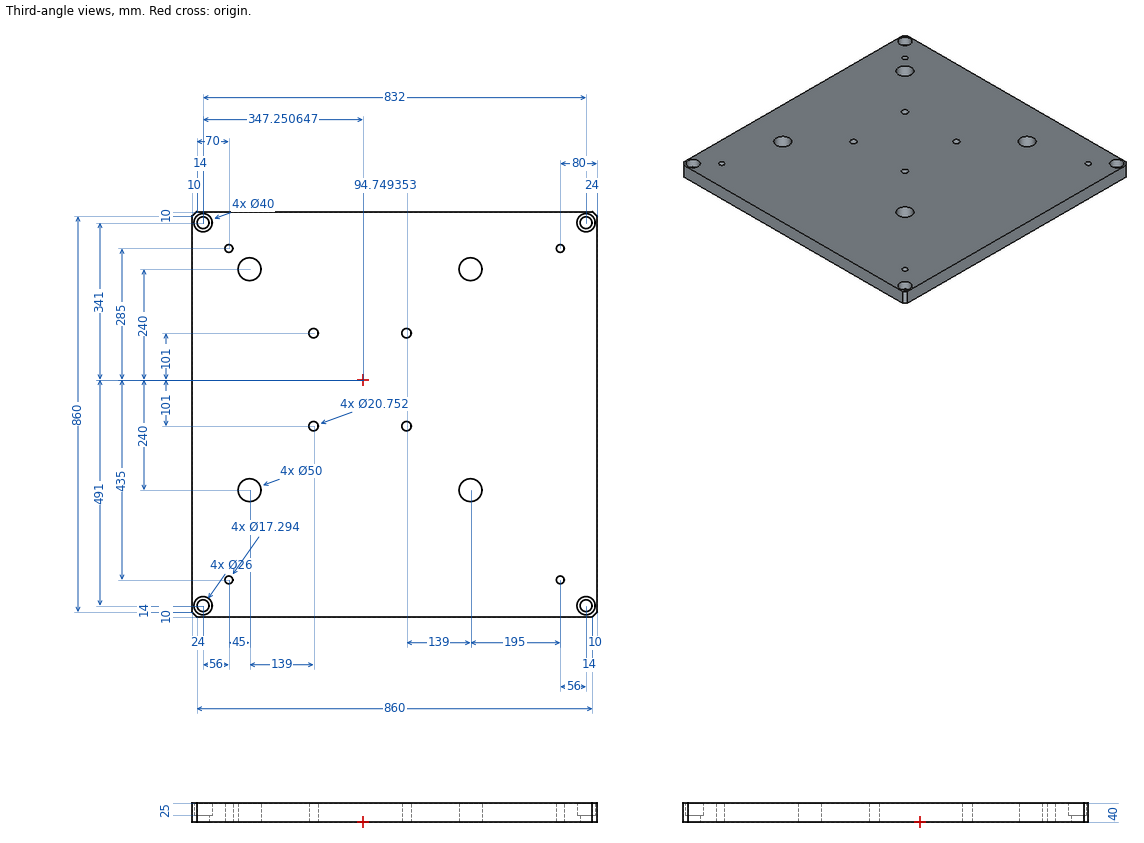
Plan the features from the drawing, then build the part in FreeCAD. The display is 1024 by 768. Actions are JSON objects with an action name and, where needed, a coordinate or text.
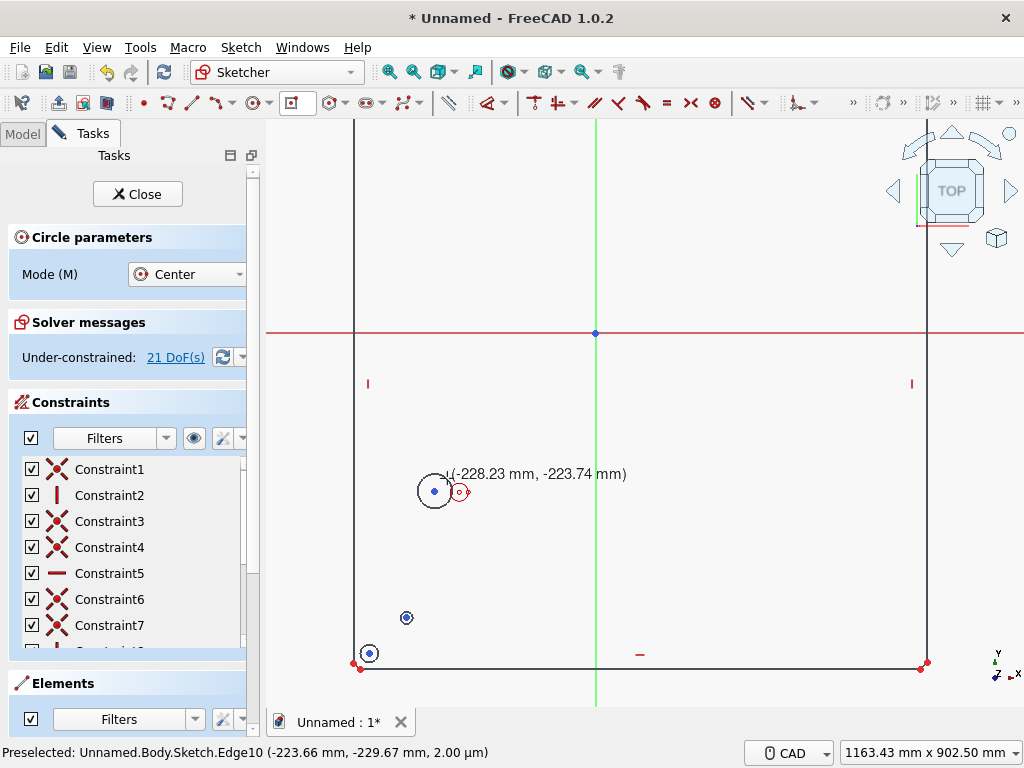
{"action": "scroll", "coordinate": [526, 399], "scroll_direction": "up", "scroll_amount": 7}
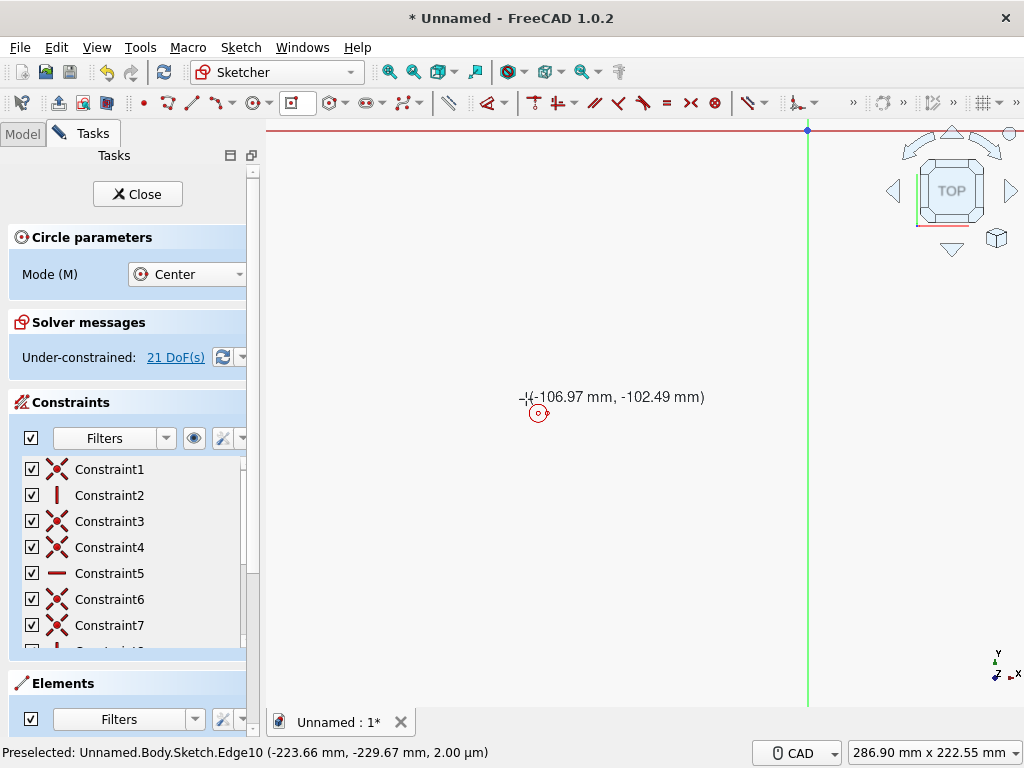
{"action": "scroll", "coordinate": [495, 430], "scroll_direction": "down", "scroll_amount": 9}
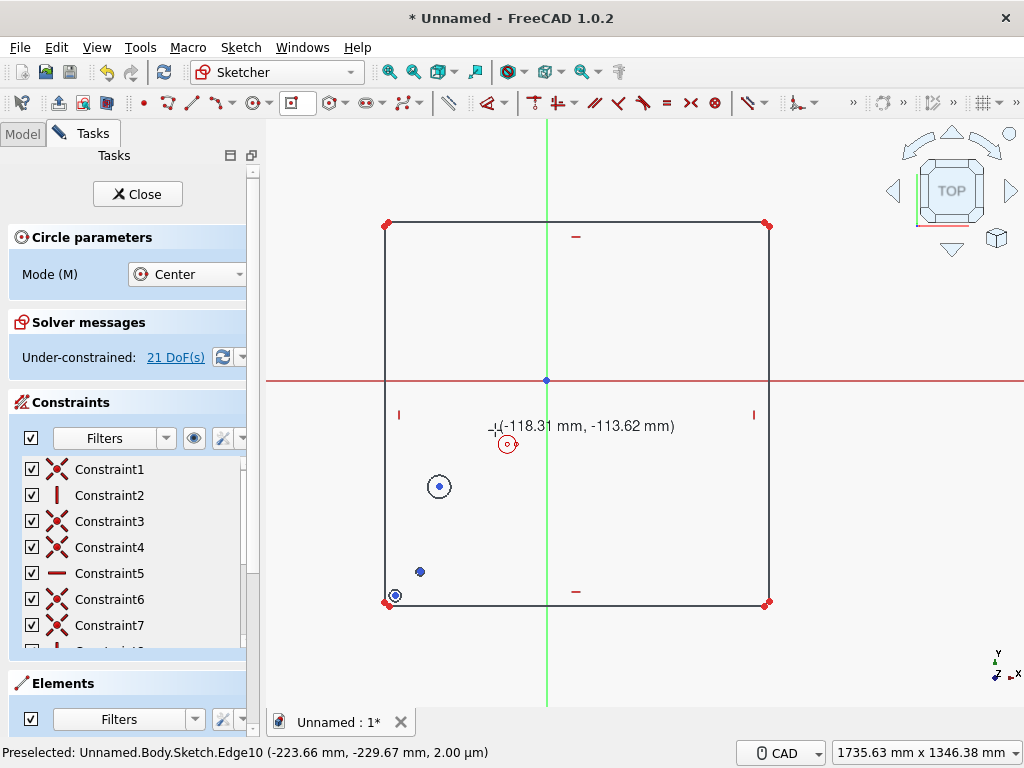
{"action": "left_click", "coordinate": [500, 425]}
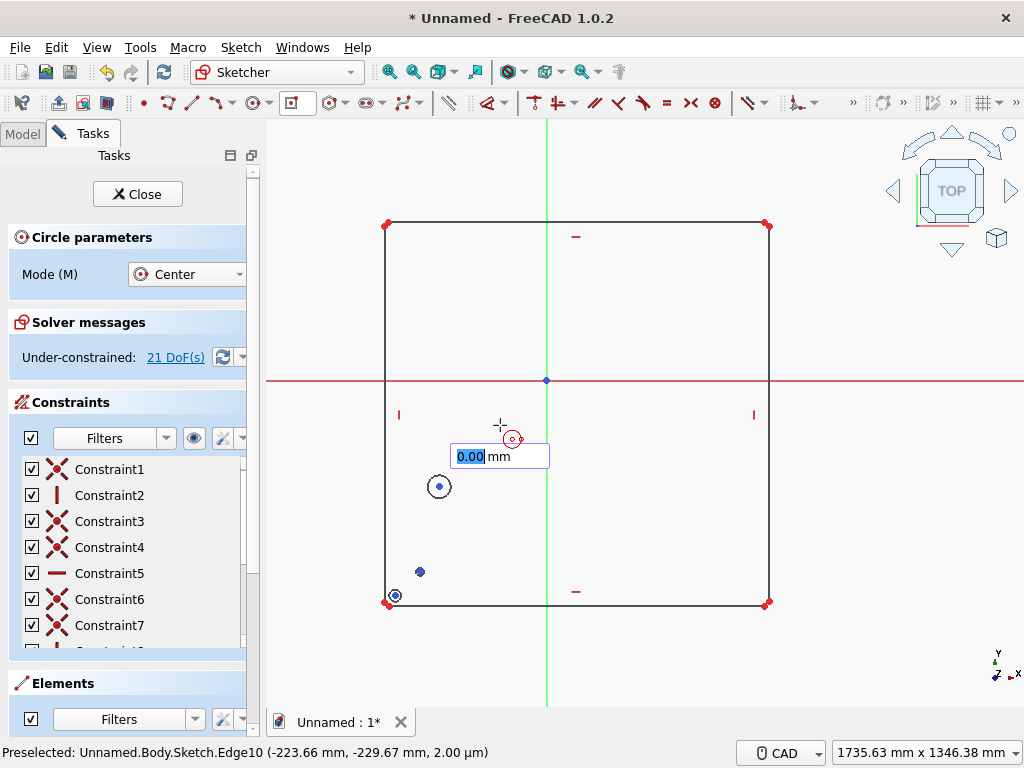
{"action": "scroll", "coordinate": [503, 422], "scroll_direction": "up", "scroll_amount": 7}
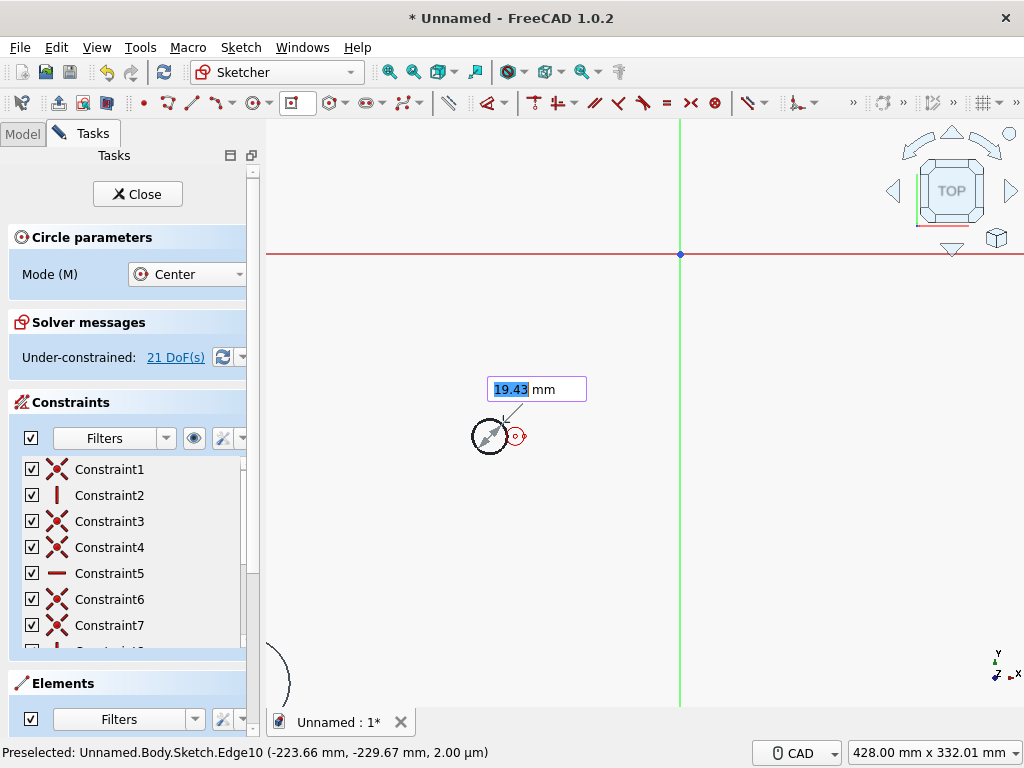
{"action": "left_click", "coordinate": [503, 420]}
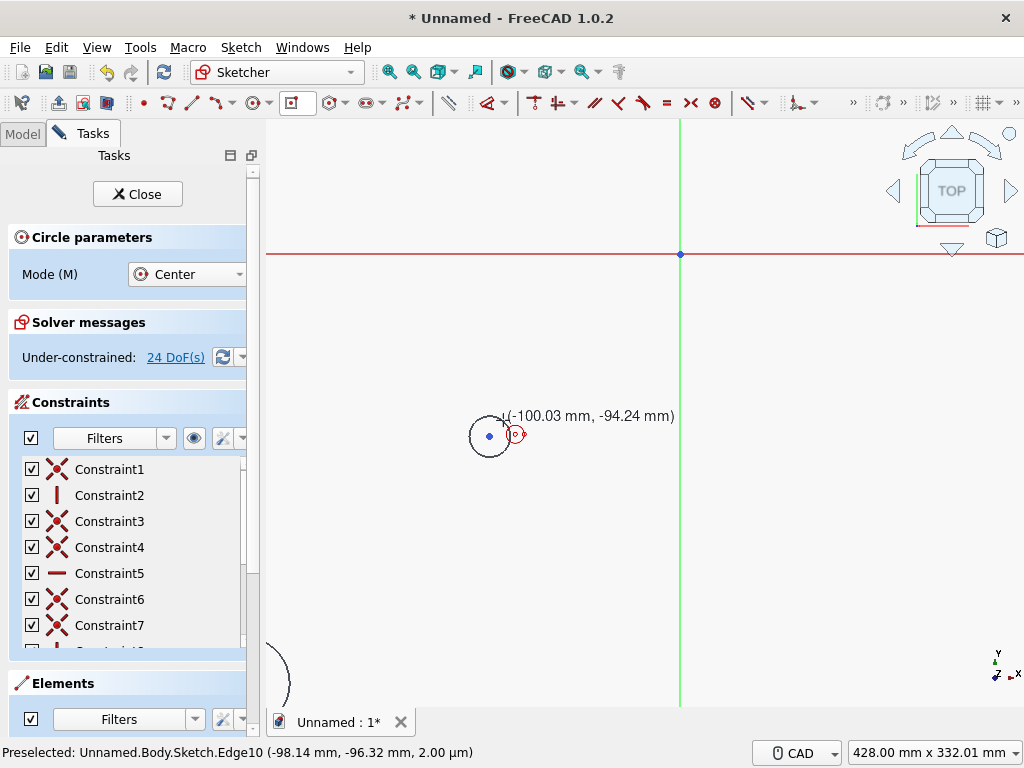
{"action": "scroll", "coordinate": [503, 422], "scroll_direction": "down", "scroll_amount": 7}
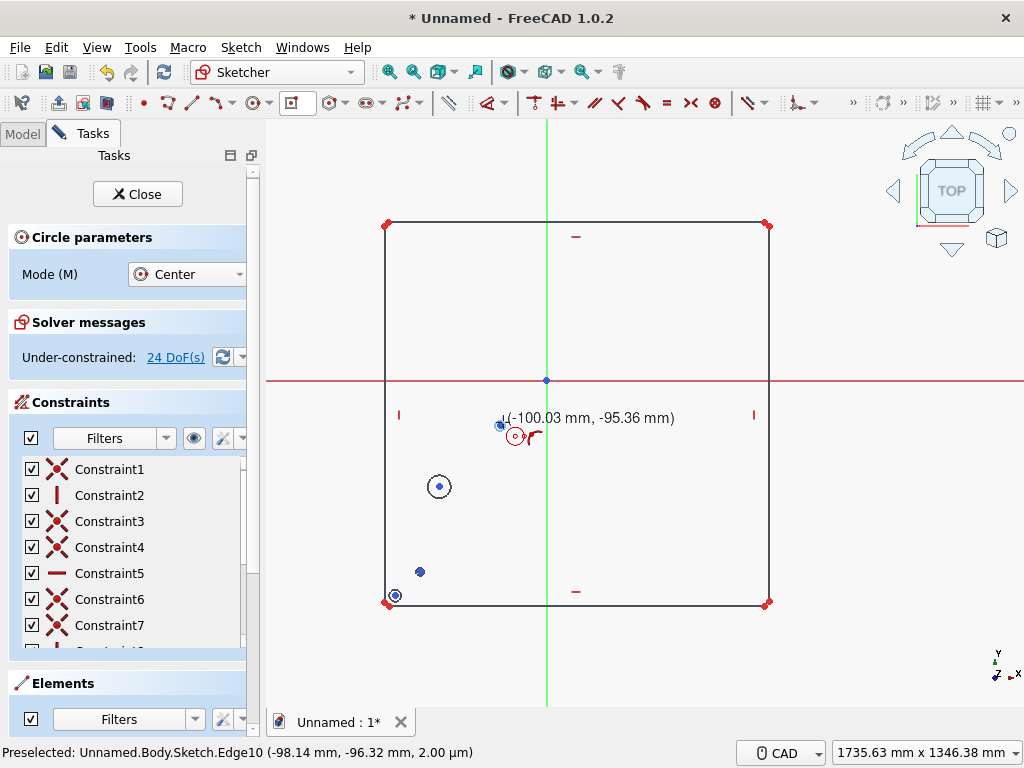
{"action": "scroll", "coordinate": [759, 595], "scroll_direction": "up", "scroll_amount": 7}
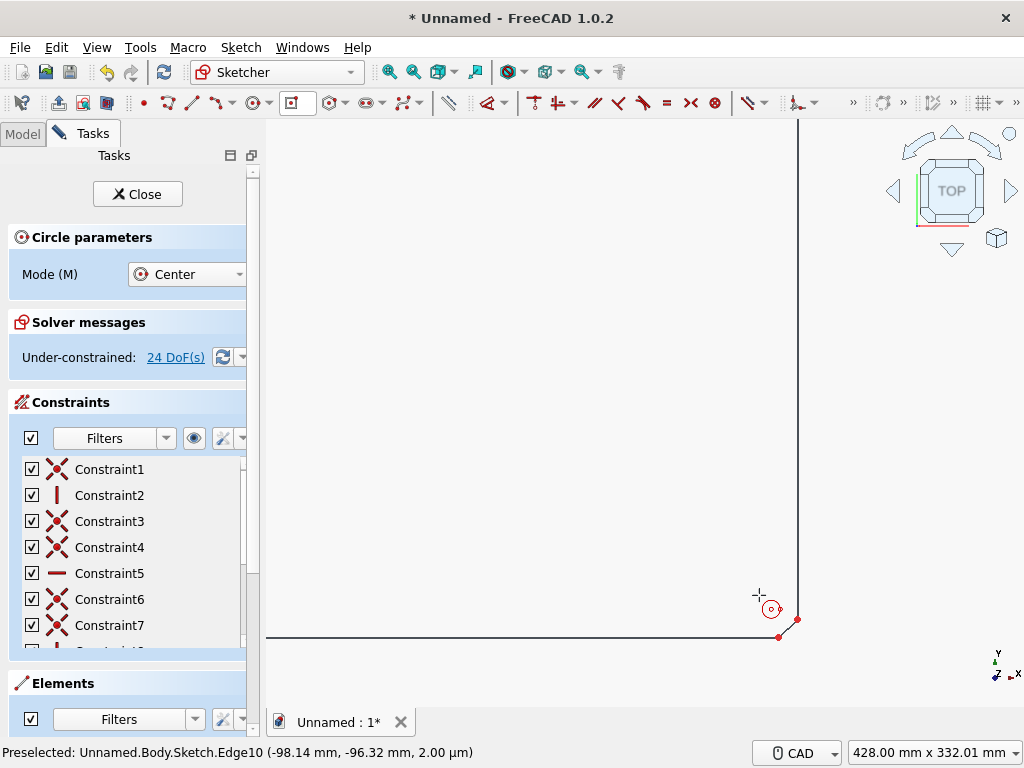
{"action": "left_click", "coordinate": [755, 594]}
{"action": "left_click", "coordinate": [772, 578]}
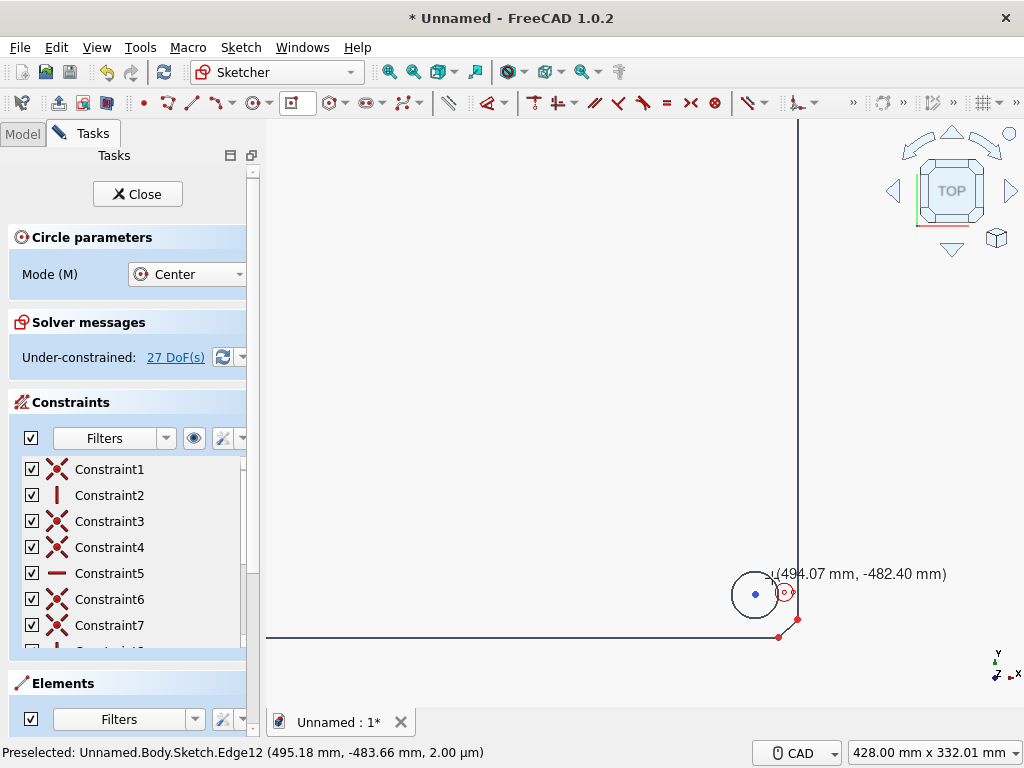
{"action": "scroll", "coordinate": [656, 495], "scroll_direction": "up", "scroll_amount": 2}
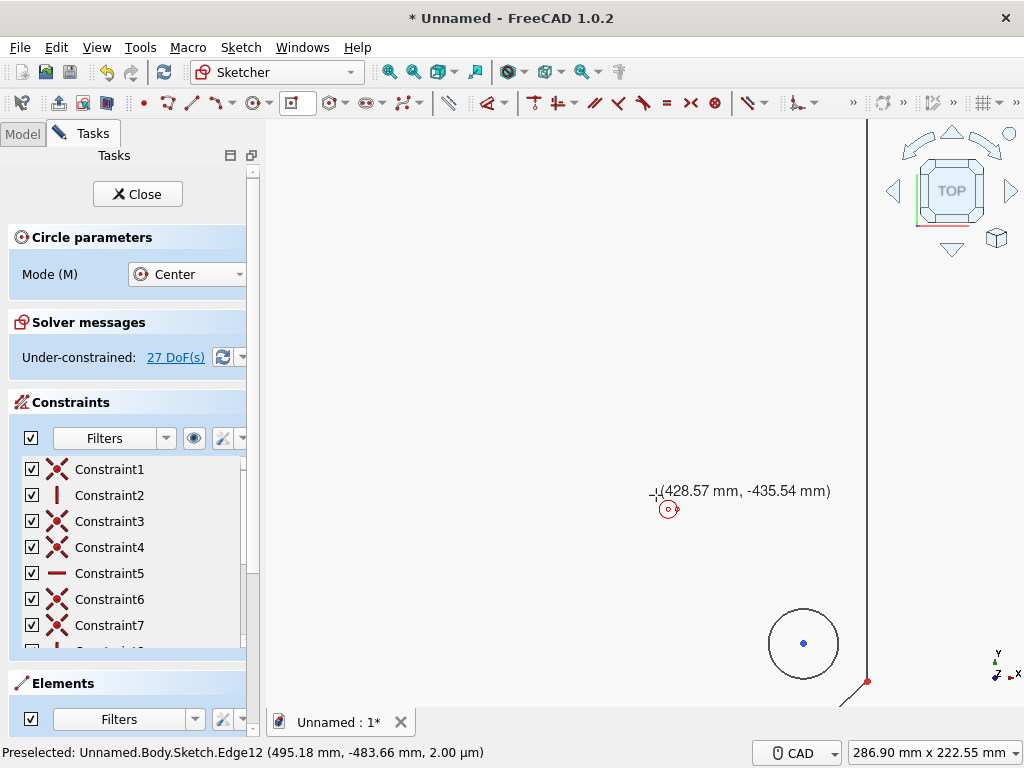
{"action": "scroll", "coordinate": [749, 585], "scroll_direction": "down", "scroll_amount": 9}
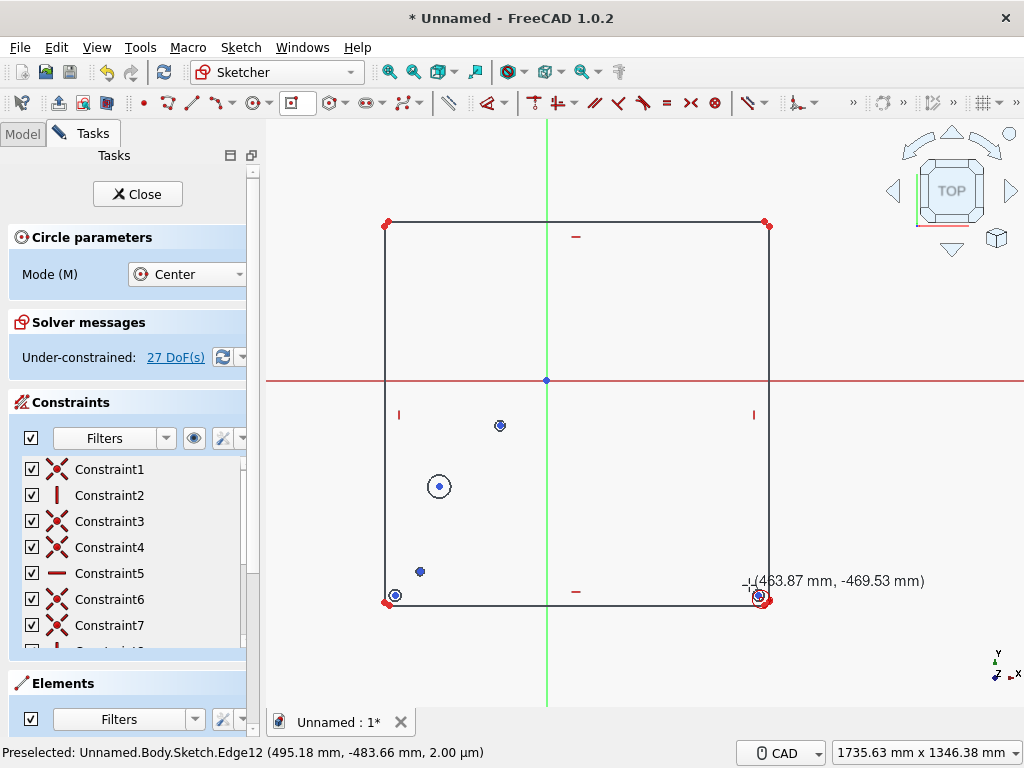
{"action": "left_click", "coordinate": [734, 571]}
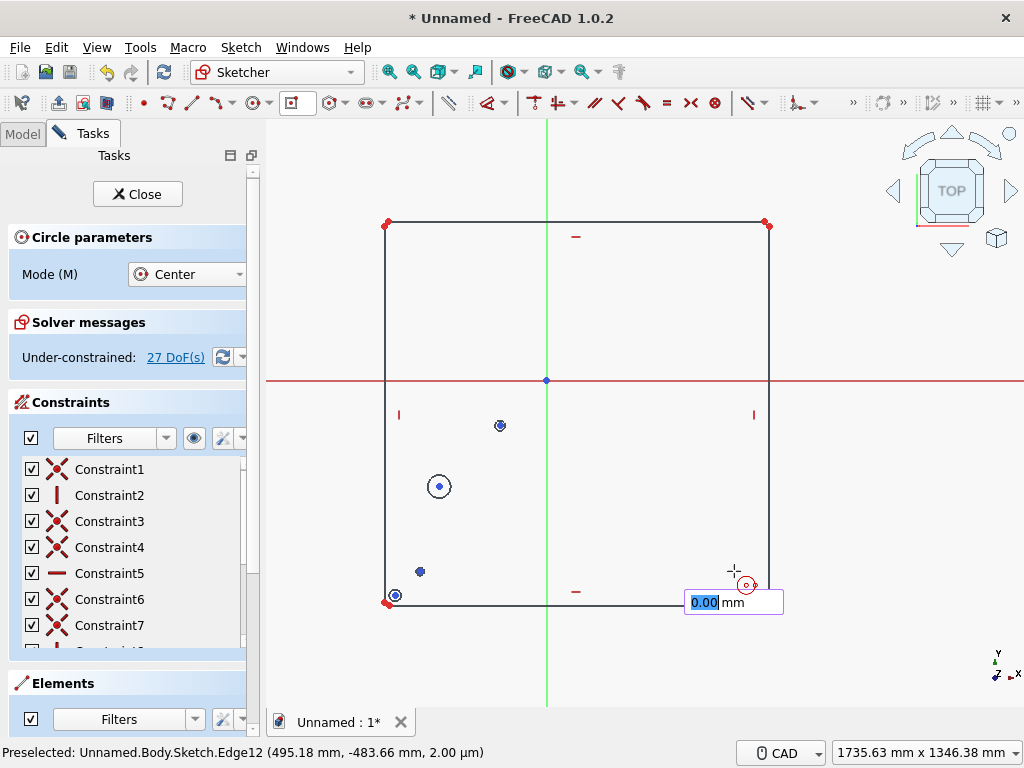
{"action": "scroll", "coordinate": [737, 568], "scroll_direction": "up", "scroll_amount": 8}